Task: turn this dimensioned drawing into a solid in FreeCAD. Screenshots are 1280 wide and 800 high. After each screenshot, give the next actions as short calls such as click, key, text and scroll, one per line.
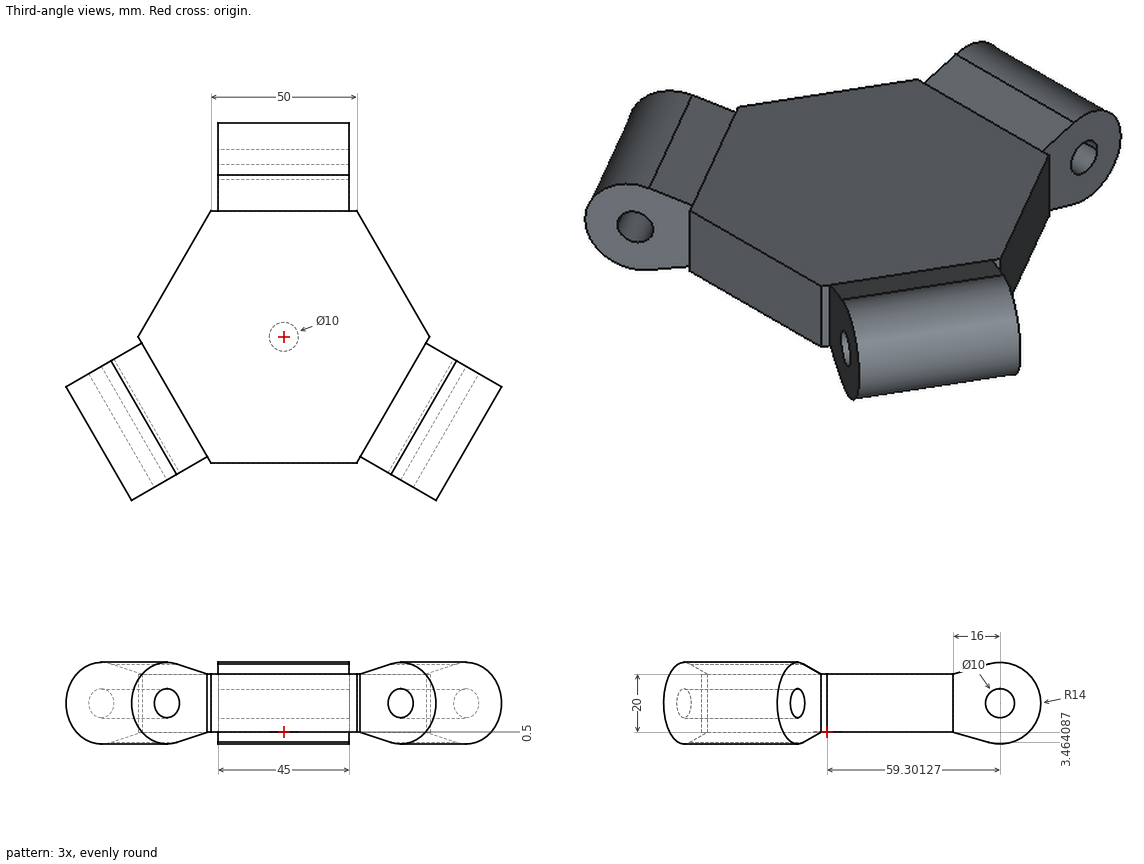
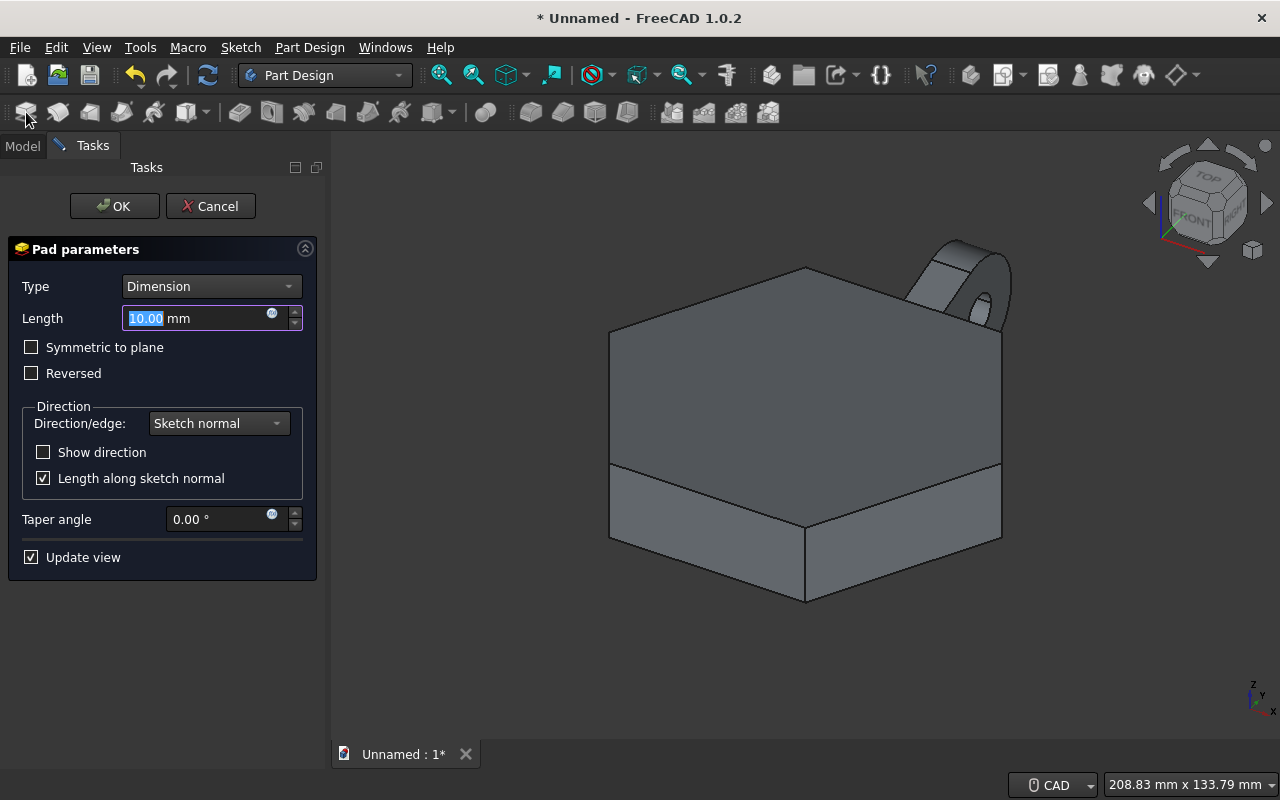
text(45)
key(Tab)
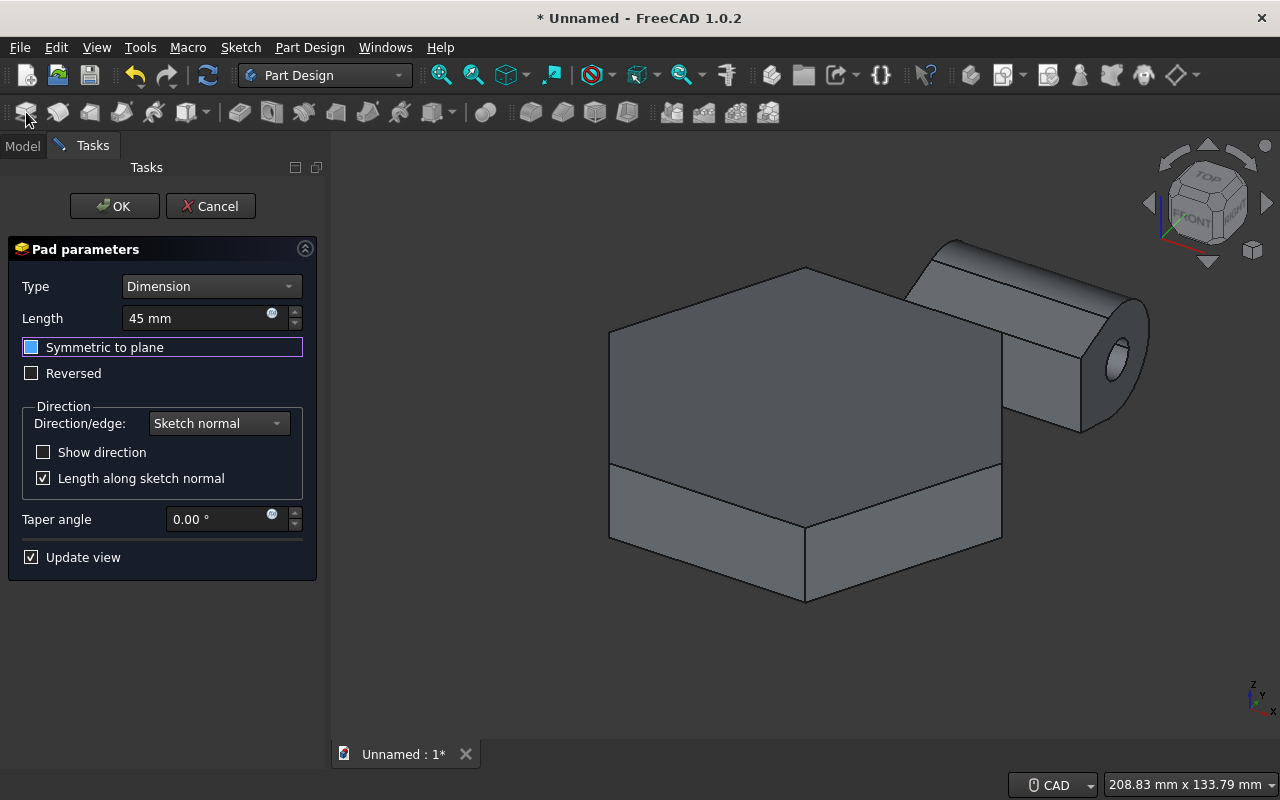
click(30, 347)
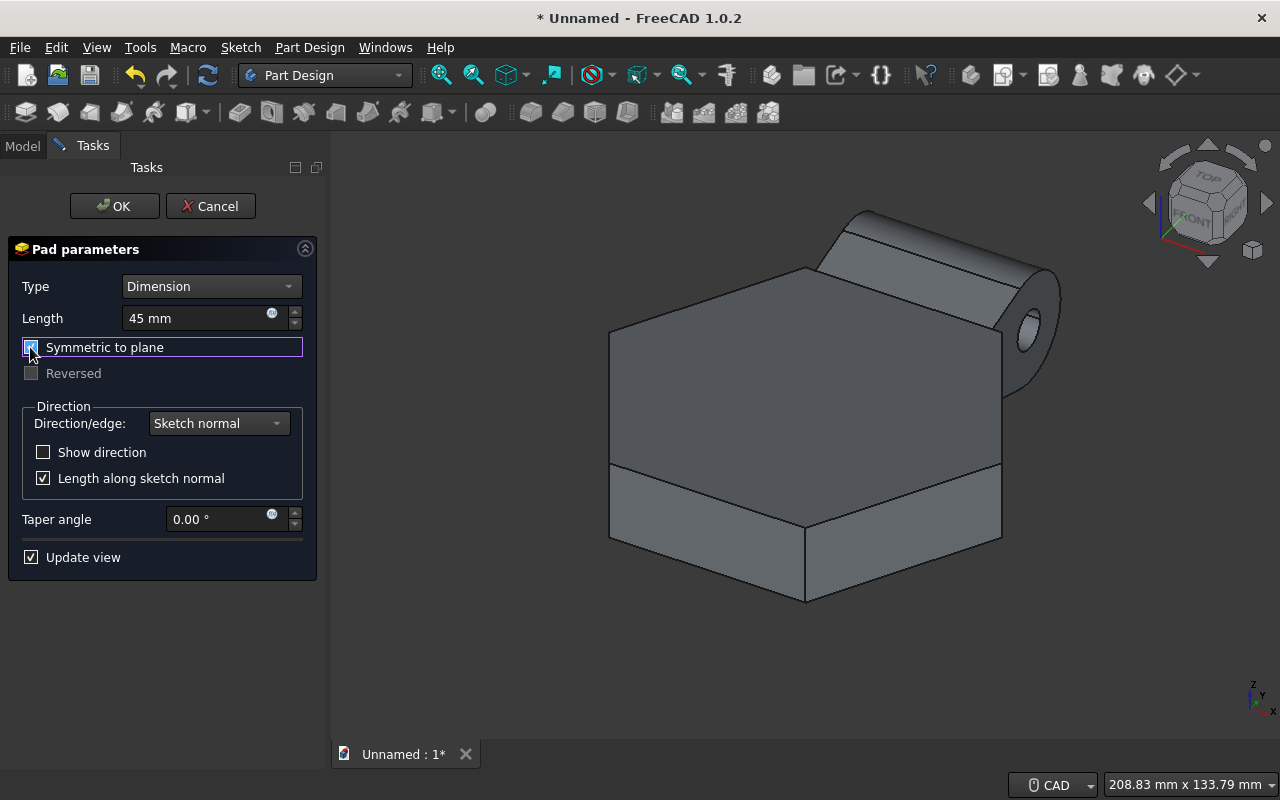
click(115, 206)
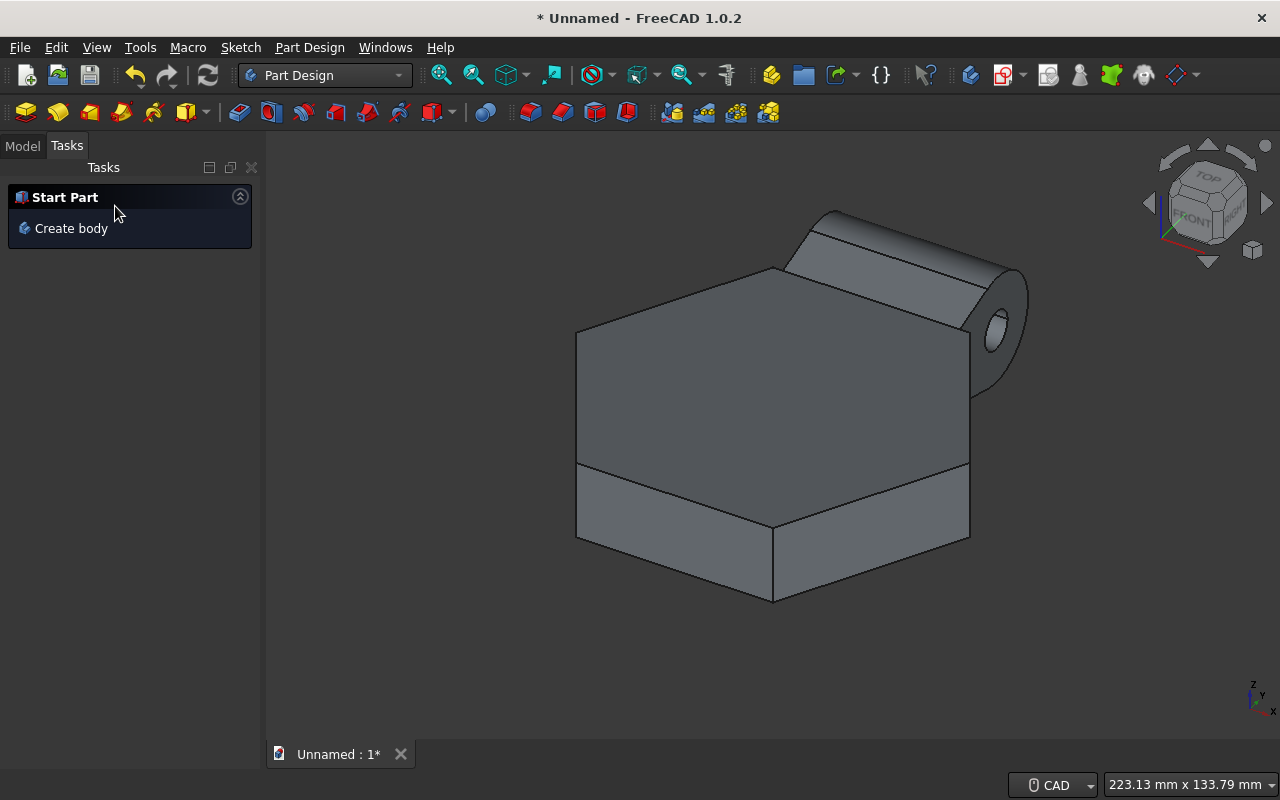
click(1004, 76)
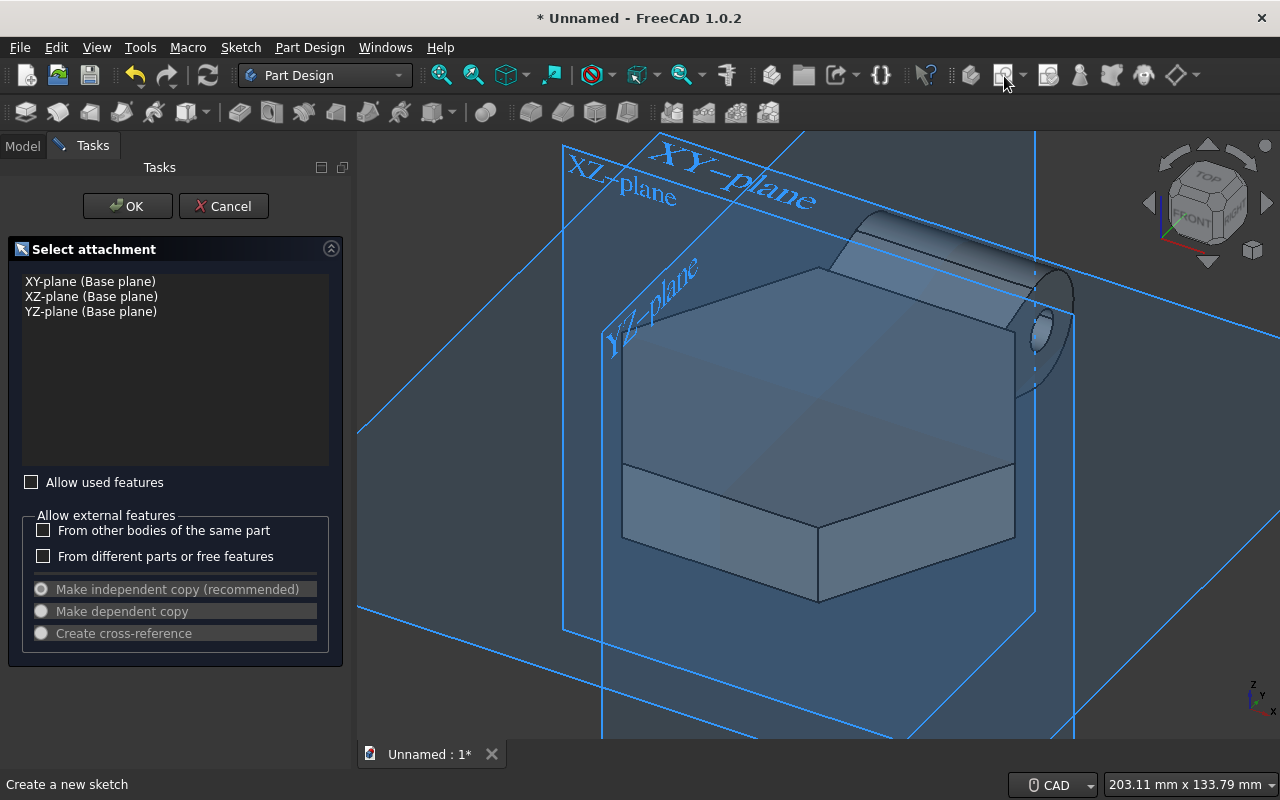
click(82, 282)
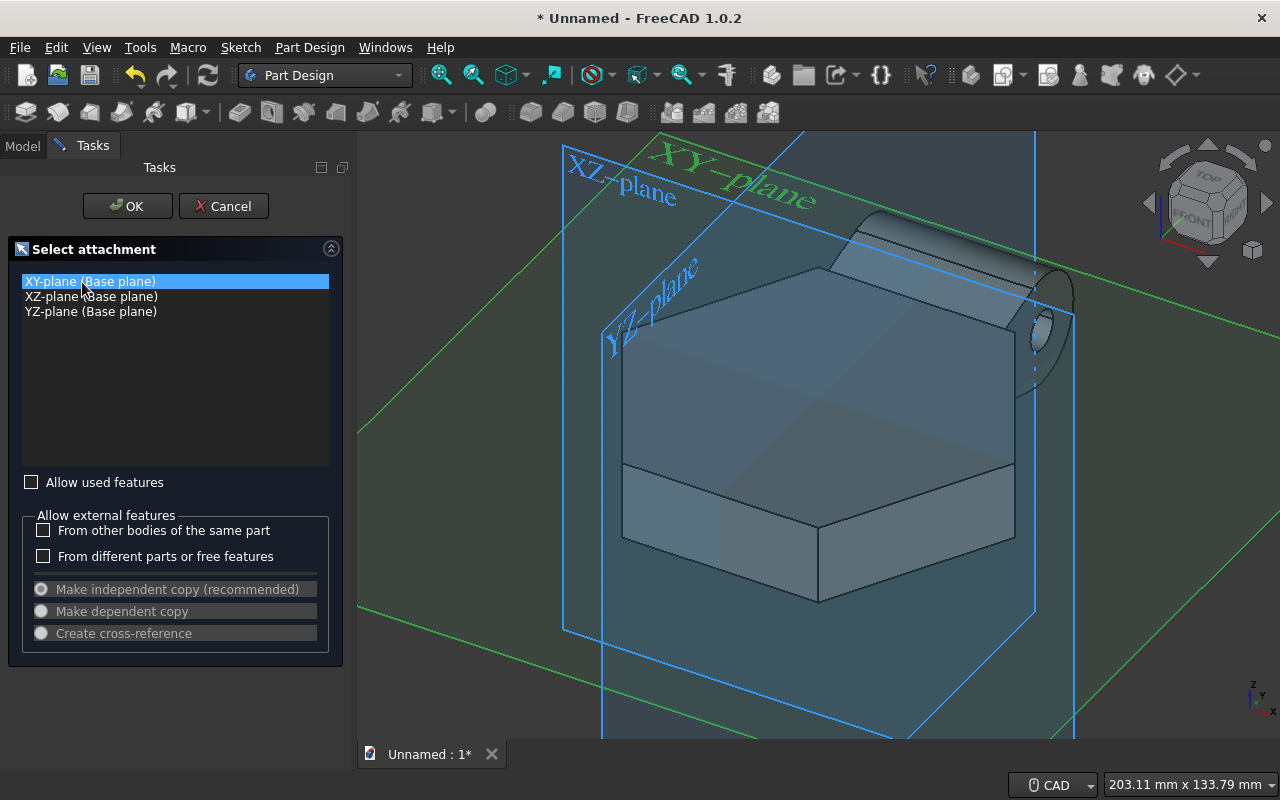
click(128, 206)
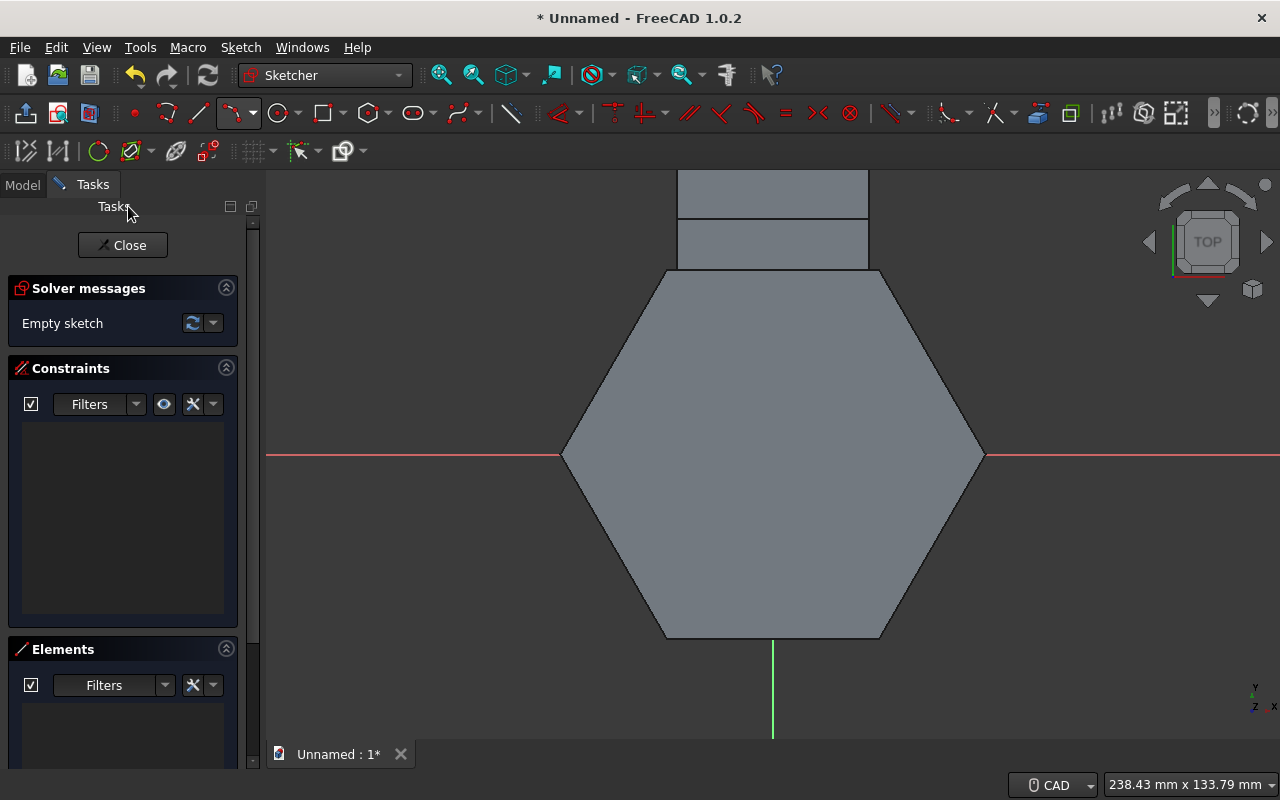
click(90, 114)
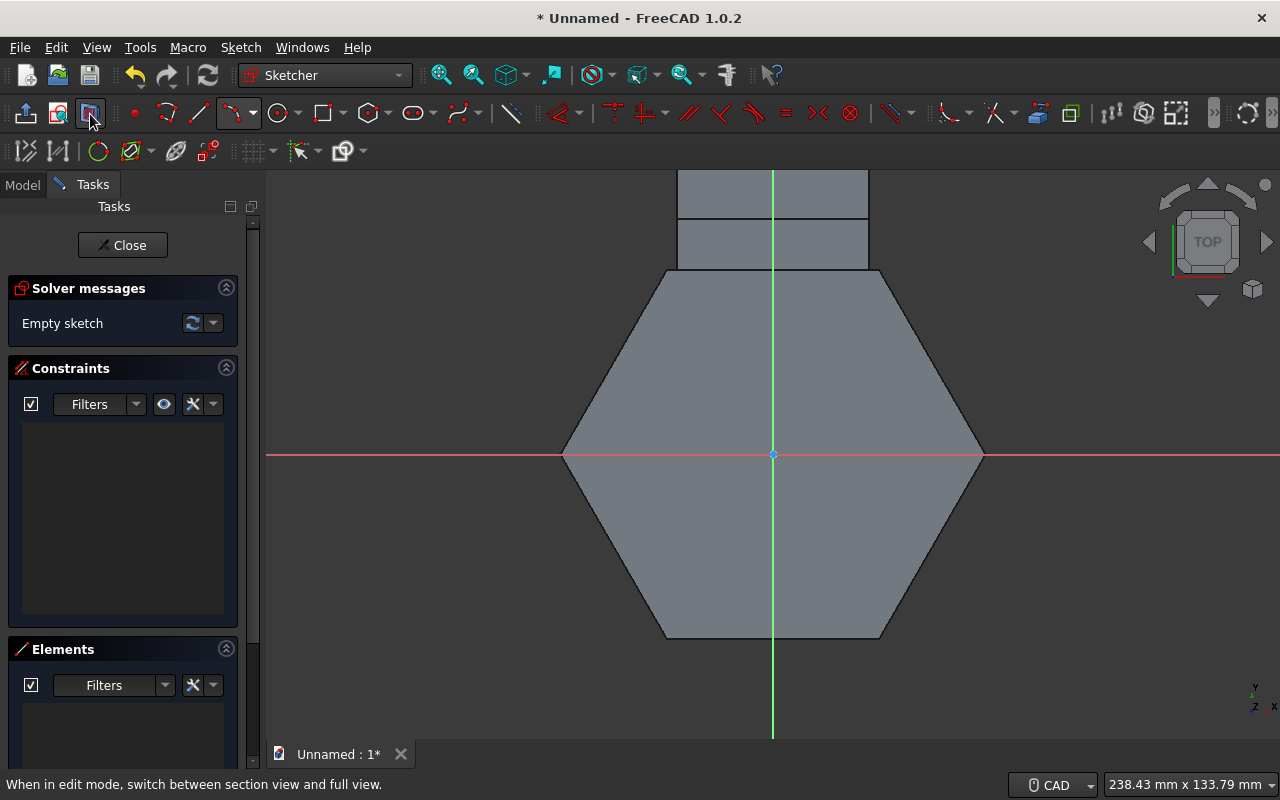
scroll(782, 454, up, 11)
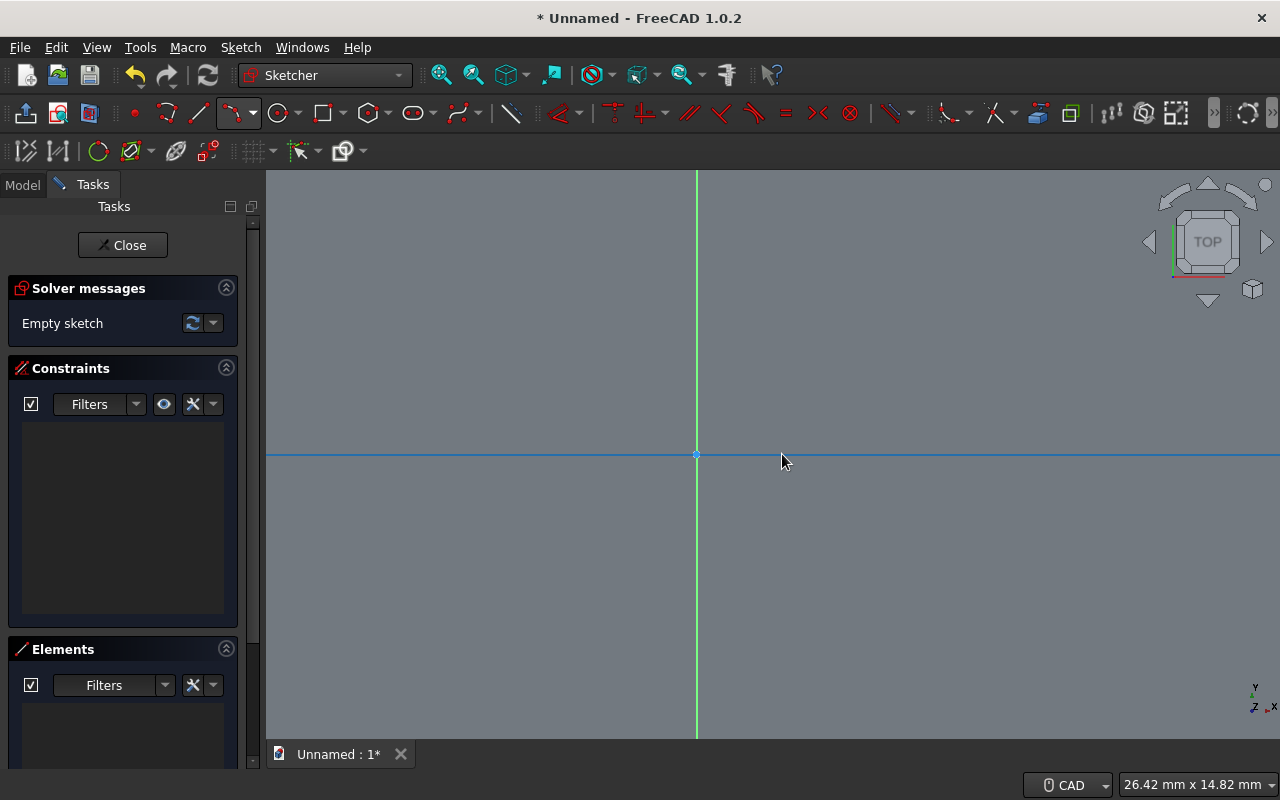
click(278, 114)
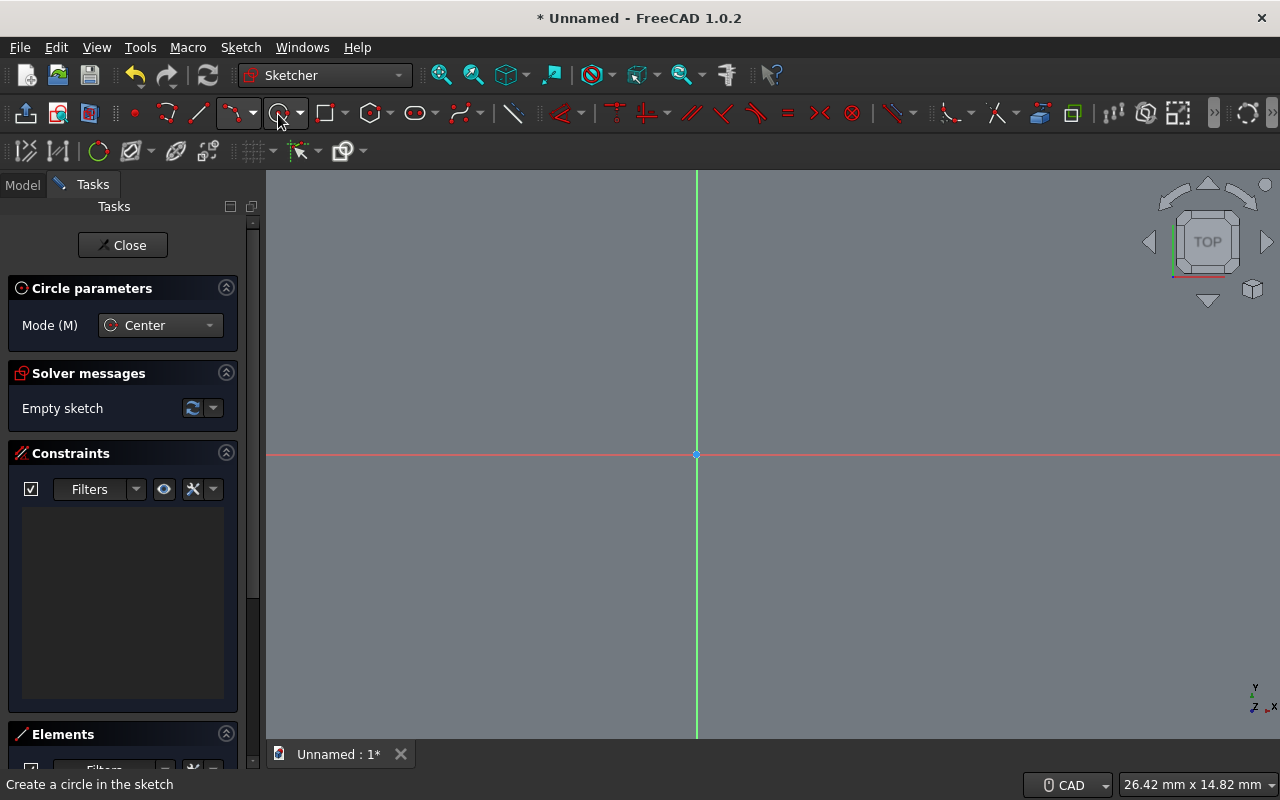
click(697, 454)
move(832, 319)